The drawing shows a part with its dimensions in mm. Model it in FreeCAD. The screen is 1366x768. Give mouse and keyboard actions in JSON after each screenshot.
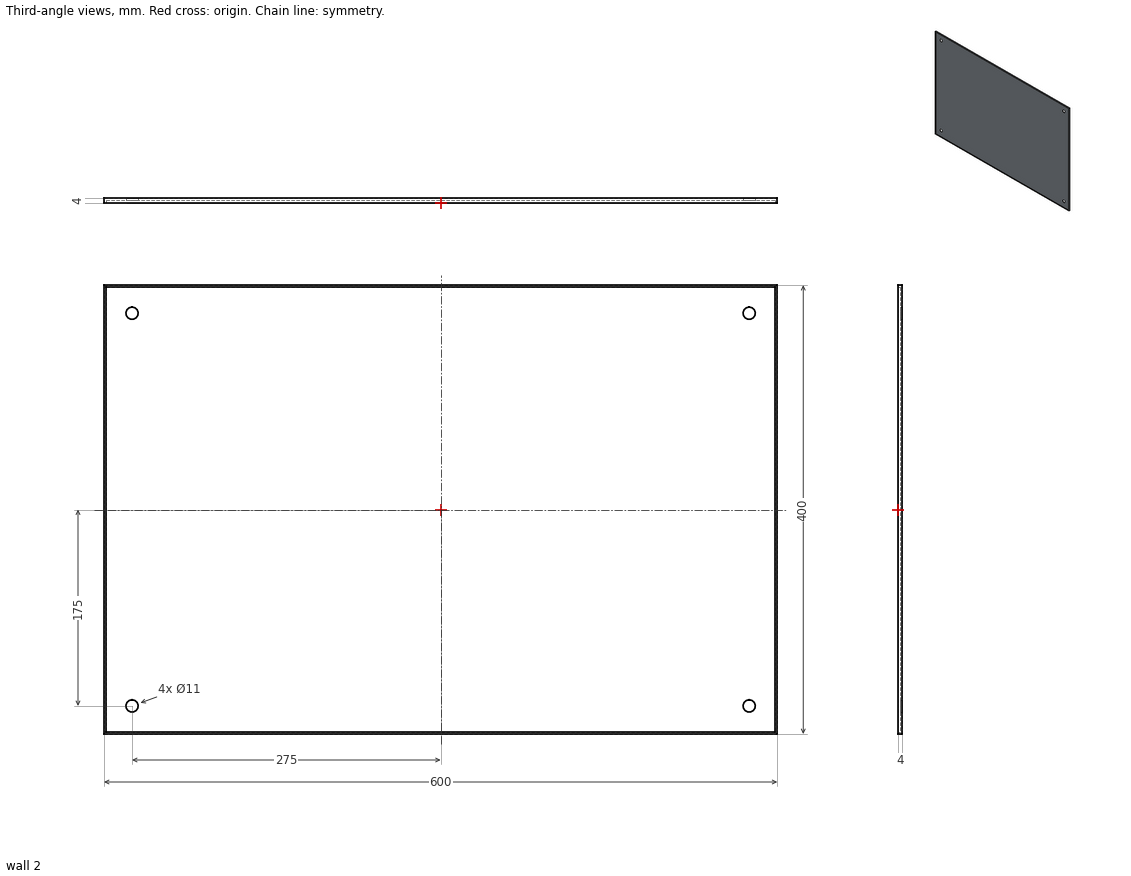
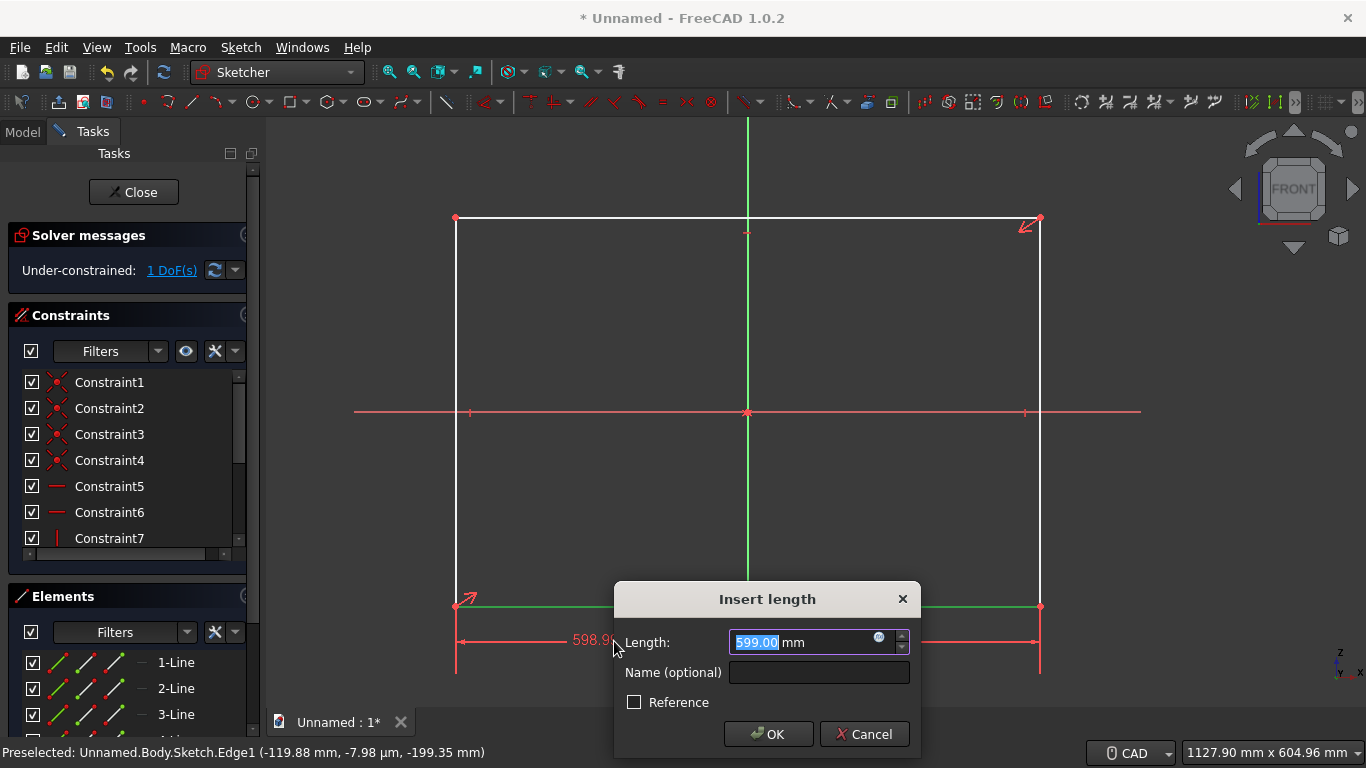
{"action": "type", "text": "600"}
{"action": "key", "text": "Return"}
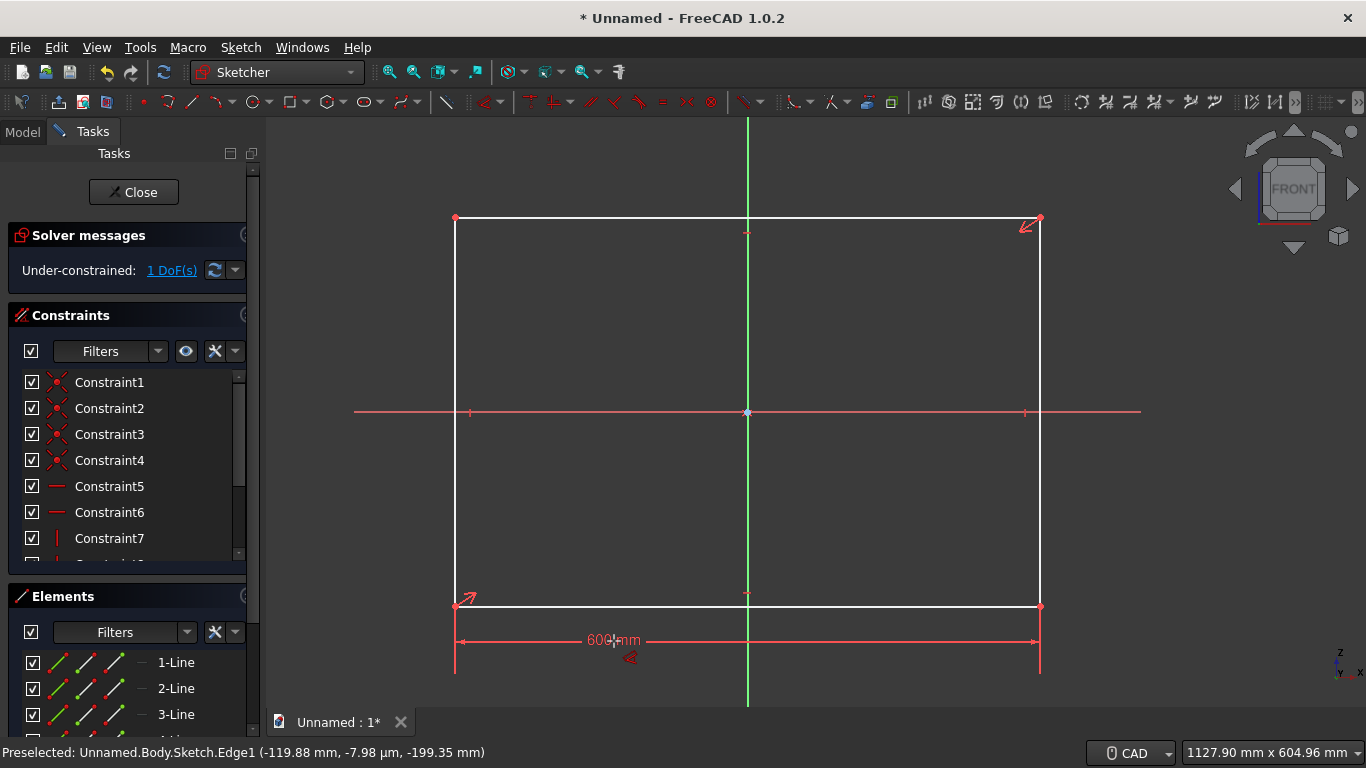
{"action": "left_click", "coordinate": [1040, 490]}
{"action": "left_click", "coordinate": [1074, 323]}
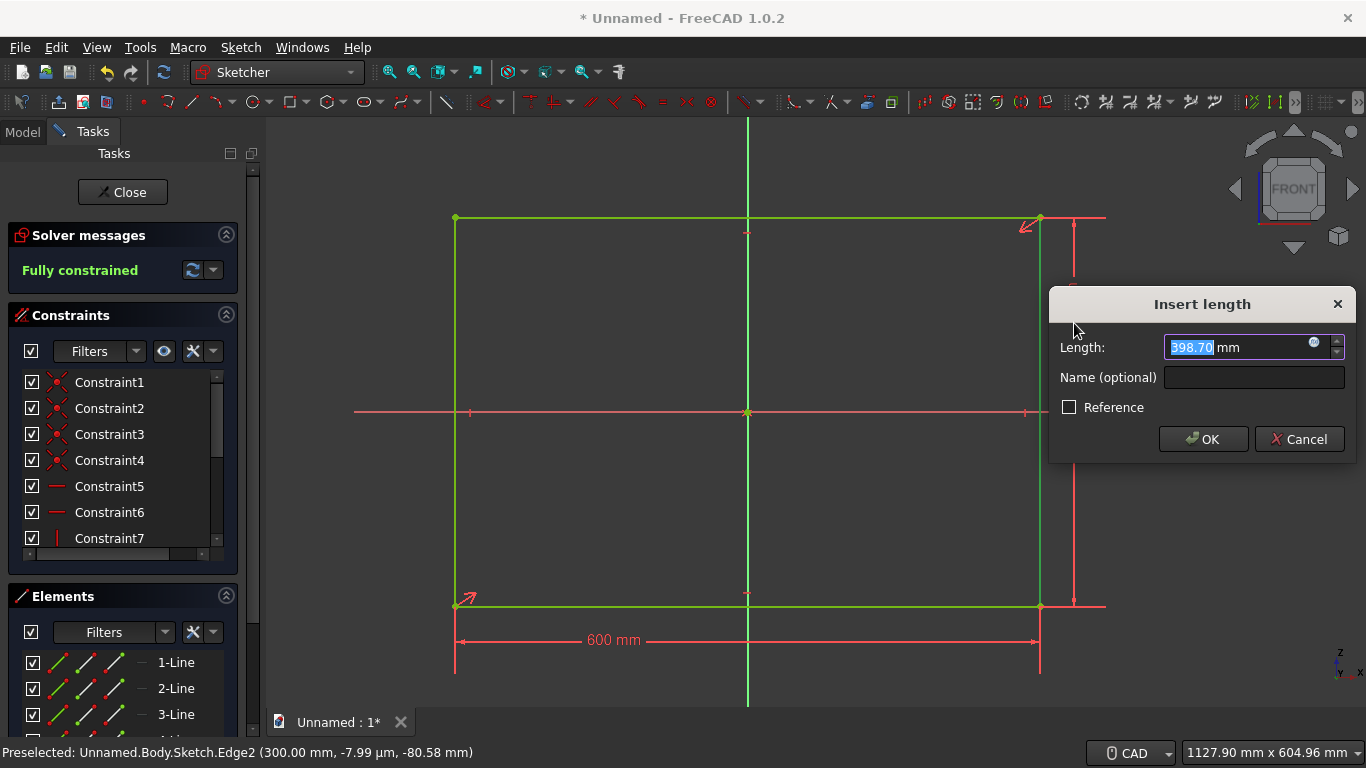
{"action": "type", "text": "400"}
{"action": "key", "text": "Return"}
{"action": "key", "text": "Escape"}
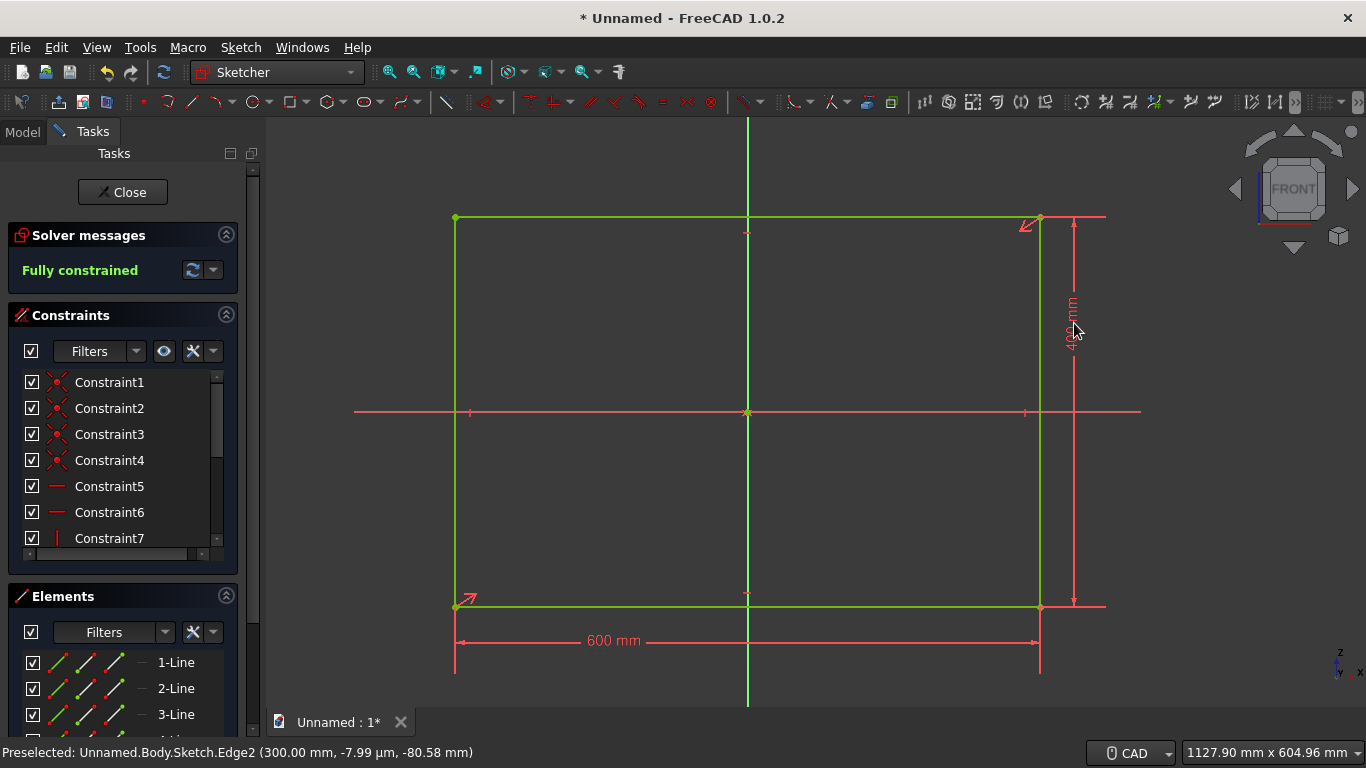
{"action": "left_click", "coordinate": [123, 192]}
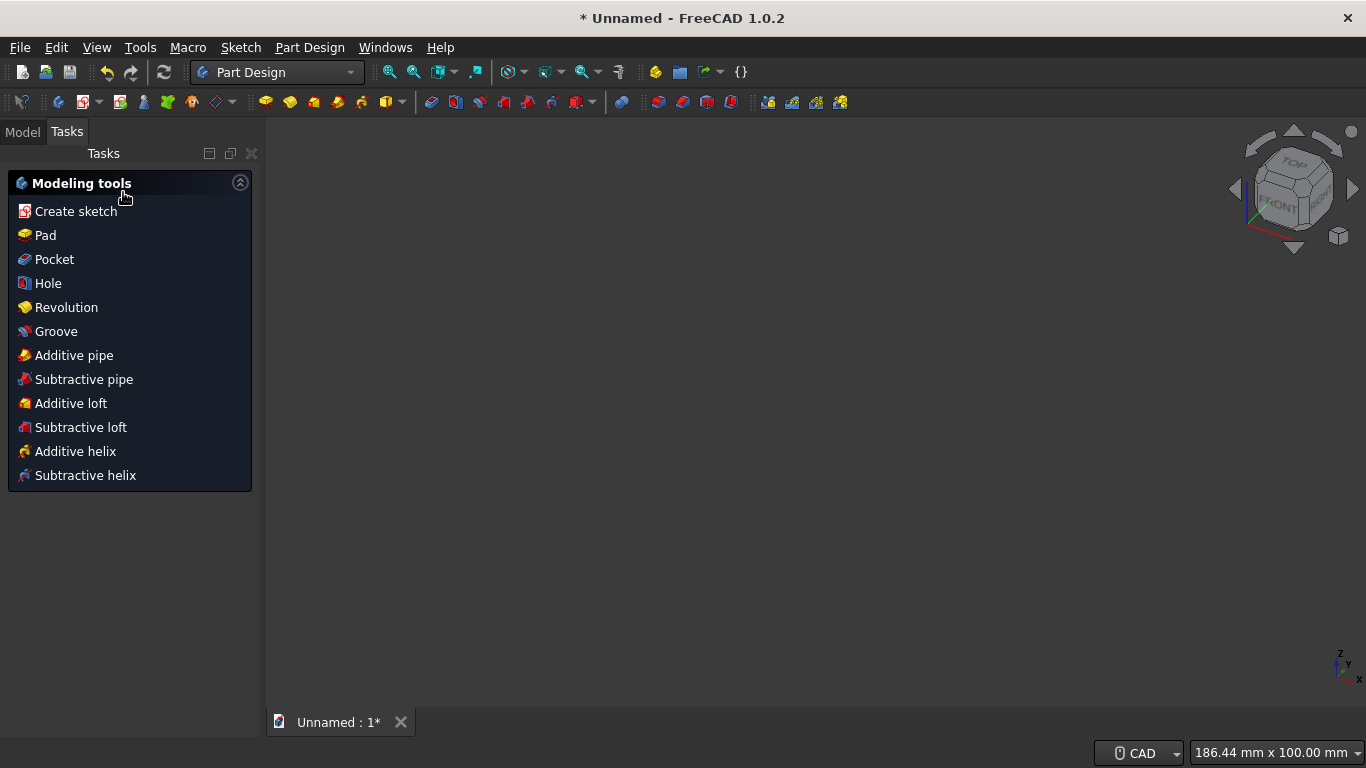
{"action": "left_click", "coordinate": [266, 102]}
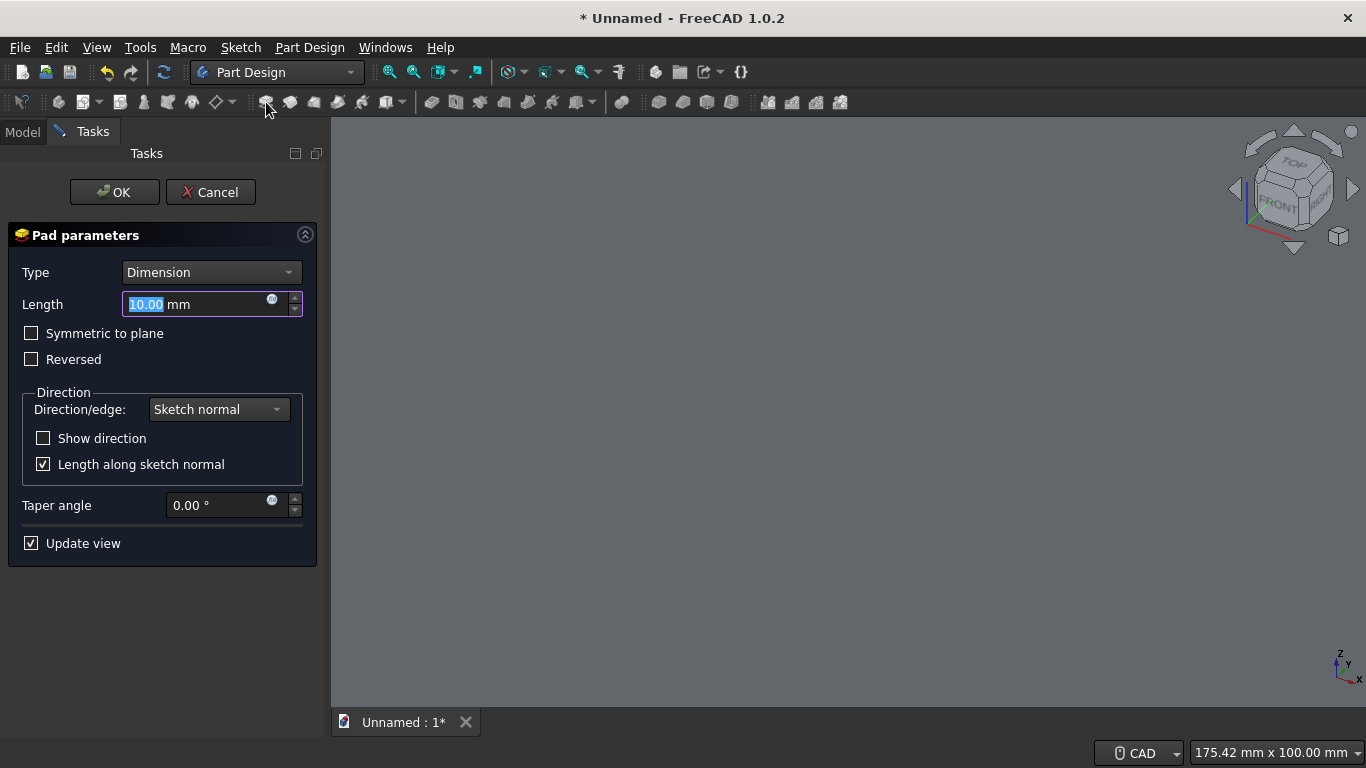
{"action": "type", "text": "4"}
{"action": "key", "text": "Tab"}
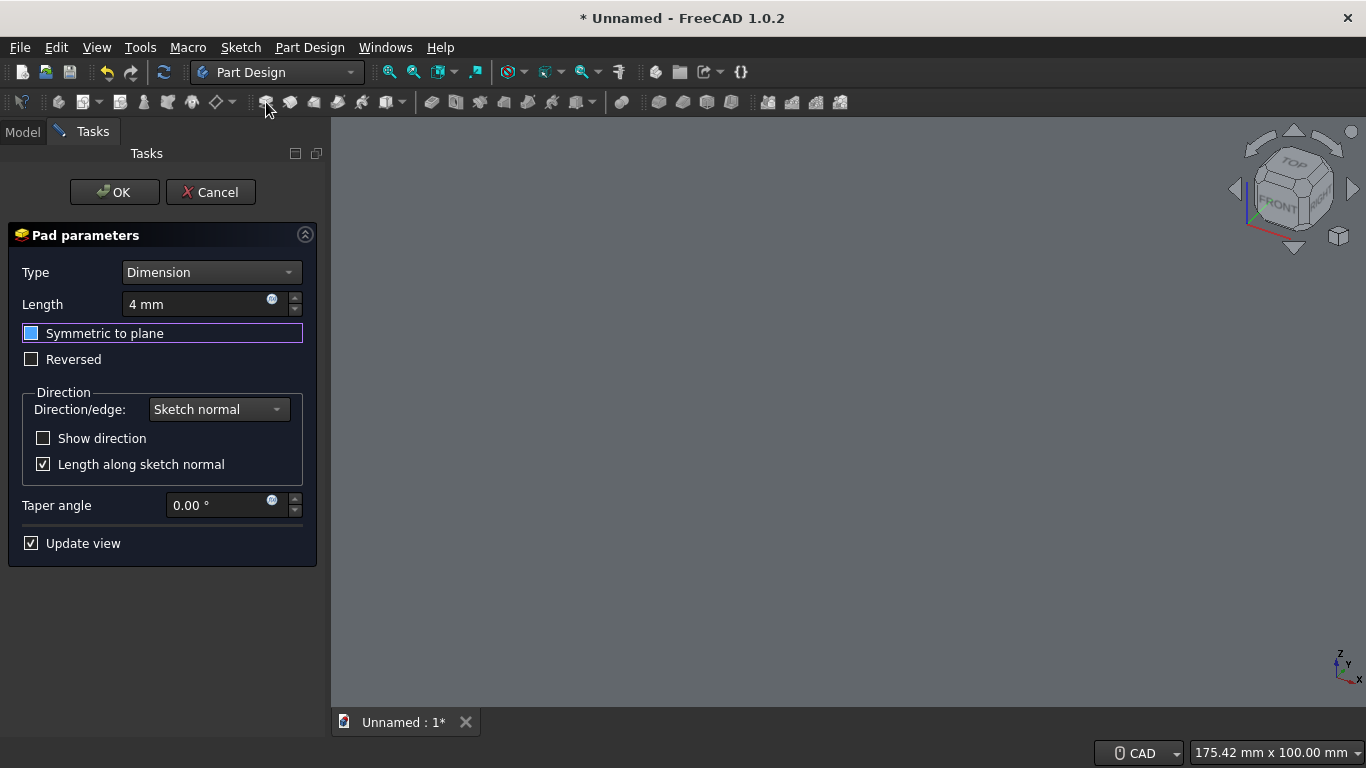
{"action": "left_click", "coordinate": [30, 359]}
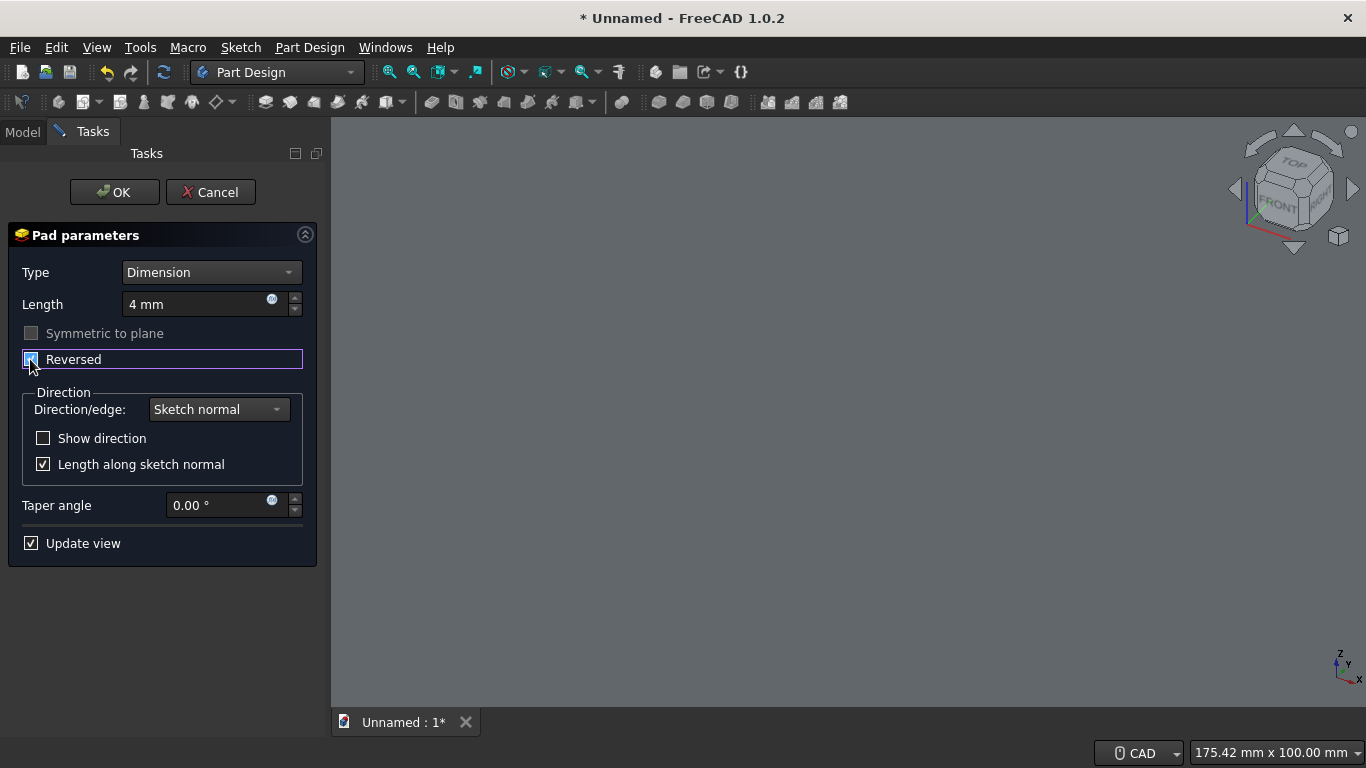
{"action": "left_click", "coordinate": [115, 192]}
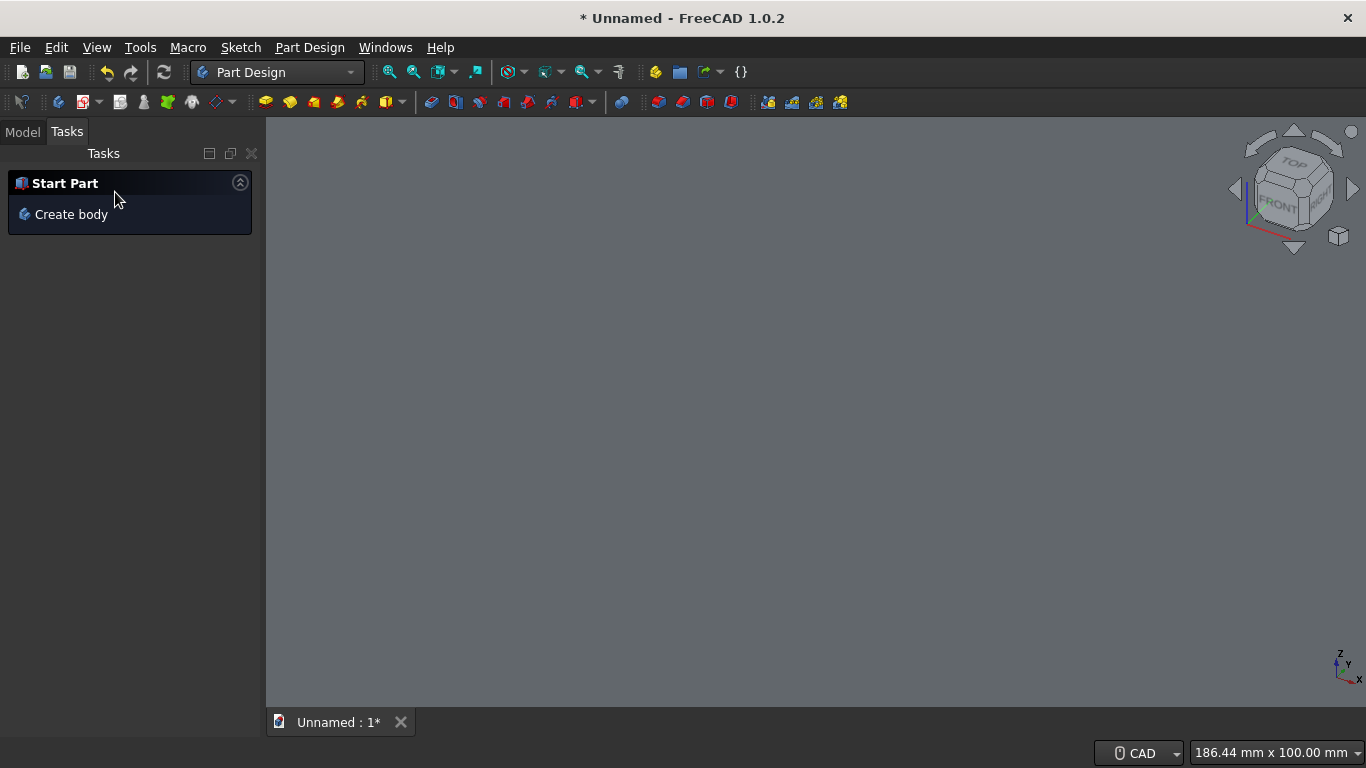
{"action": "key", "text": "v f"}